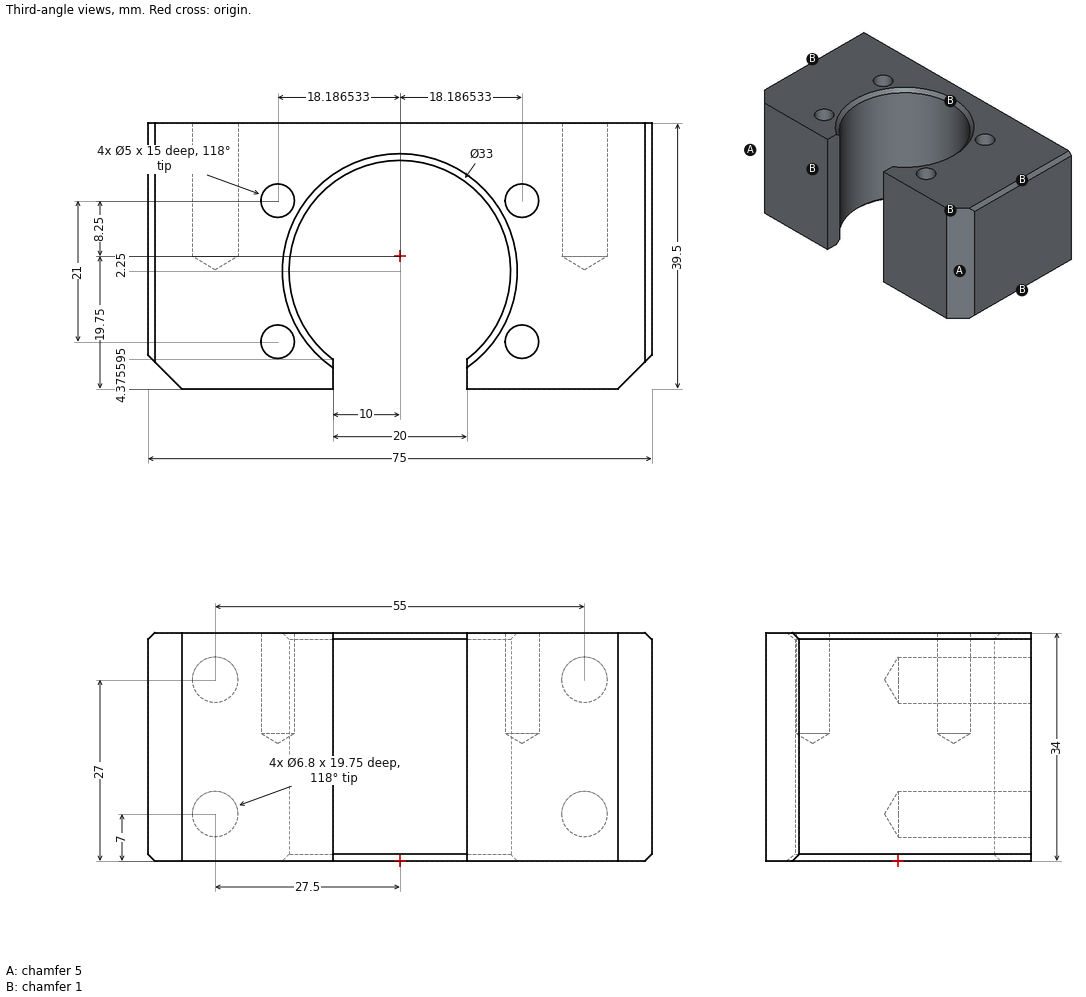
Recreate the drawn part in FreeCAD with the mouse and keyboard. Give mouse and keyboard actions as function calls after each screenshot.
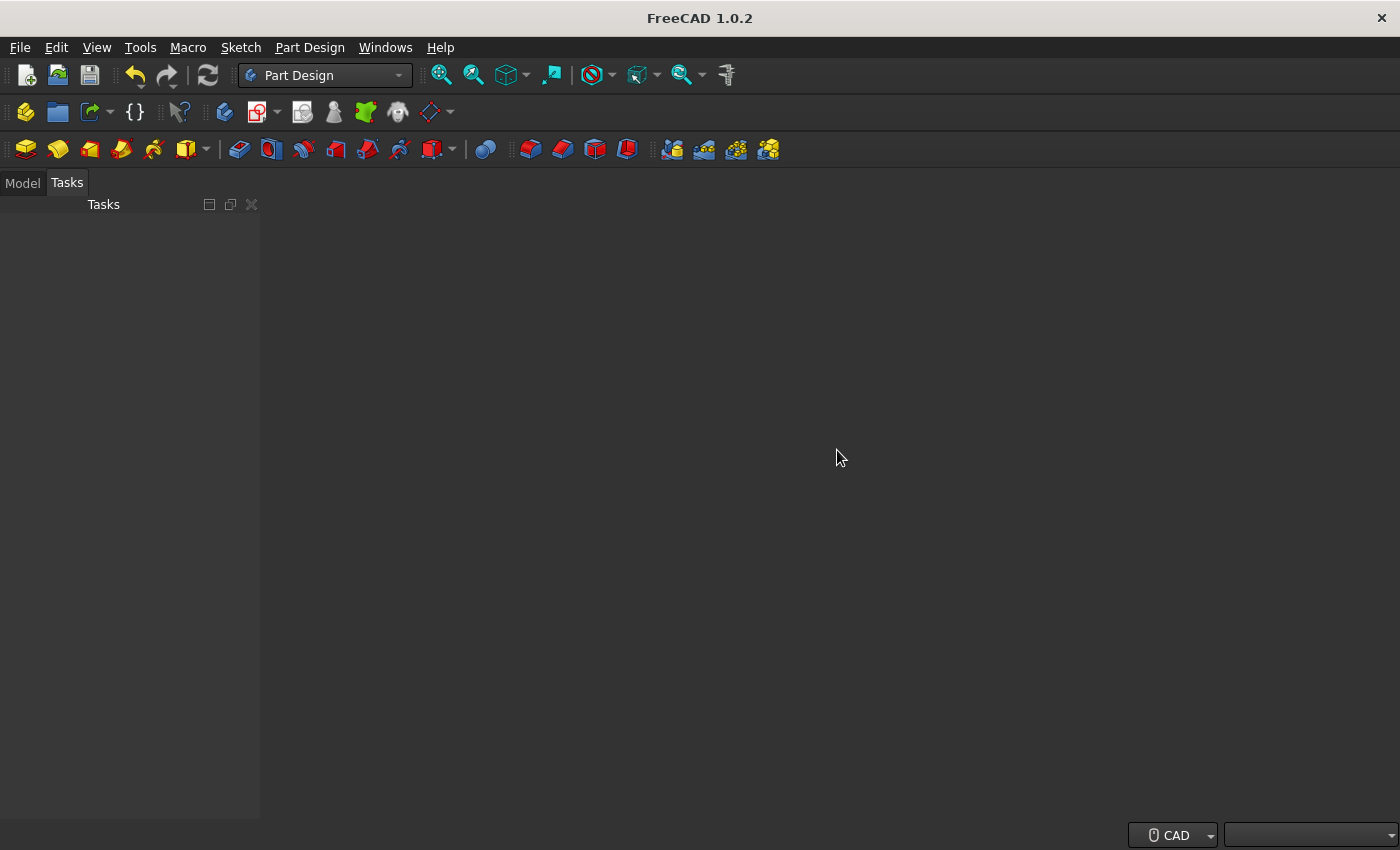
click(26, 76)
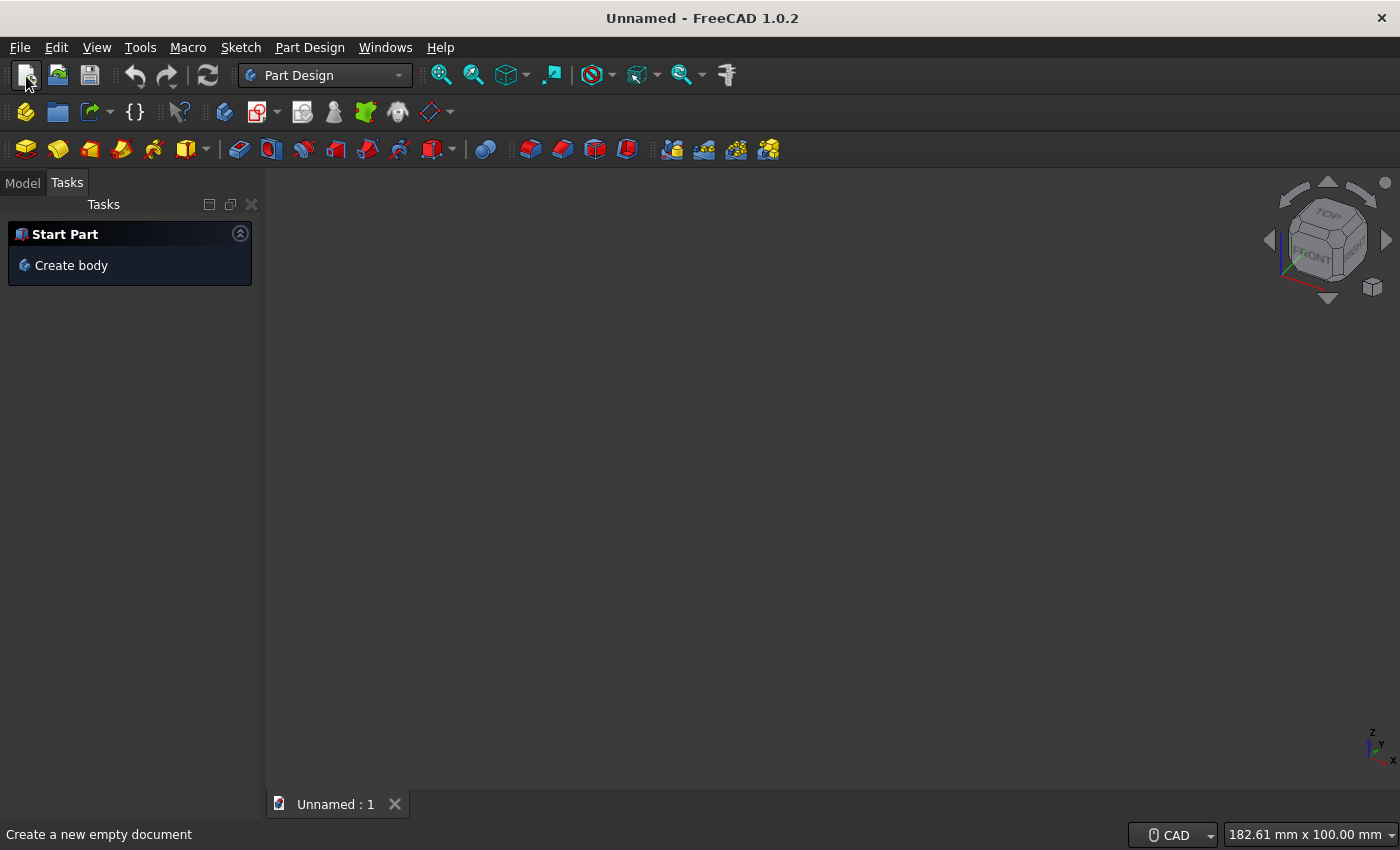
click(258, 112)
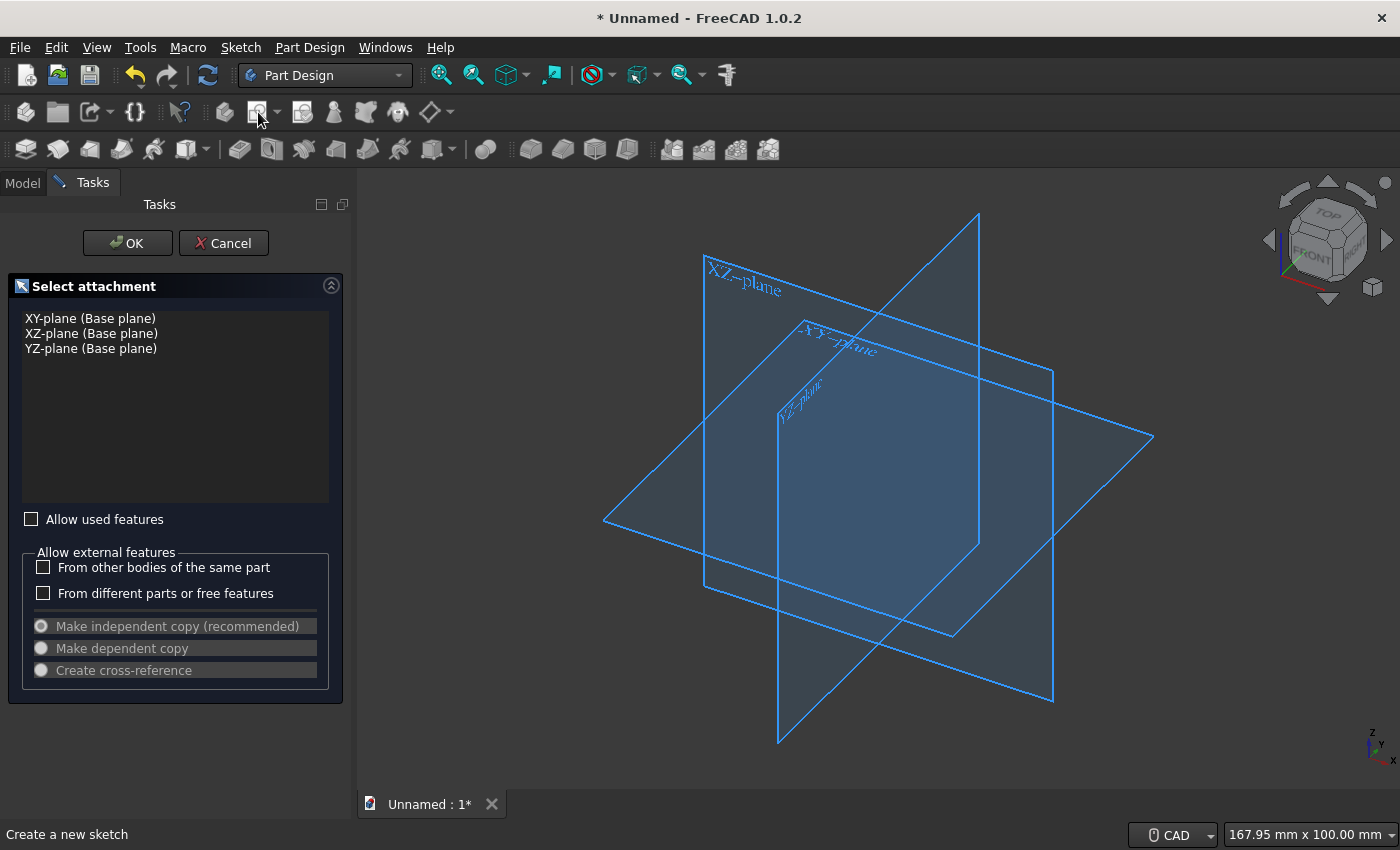
click(82, 318)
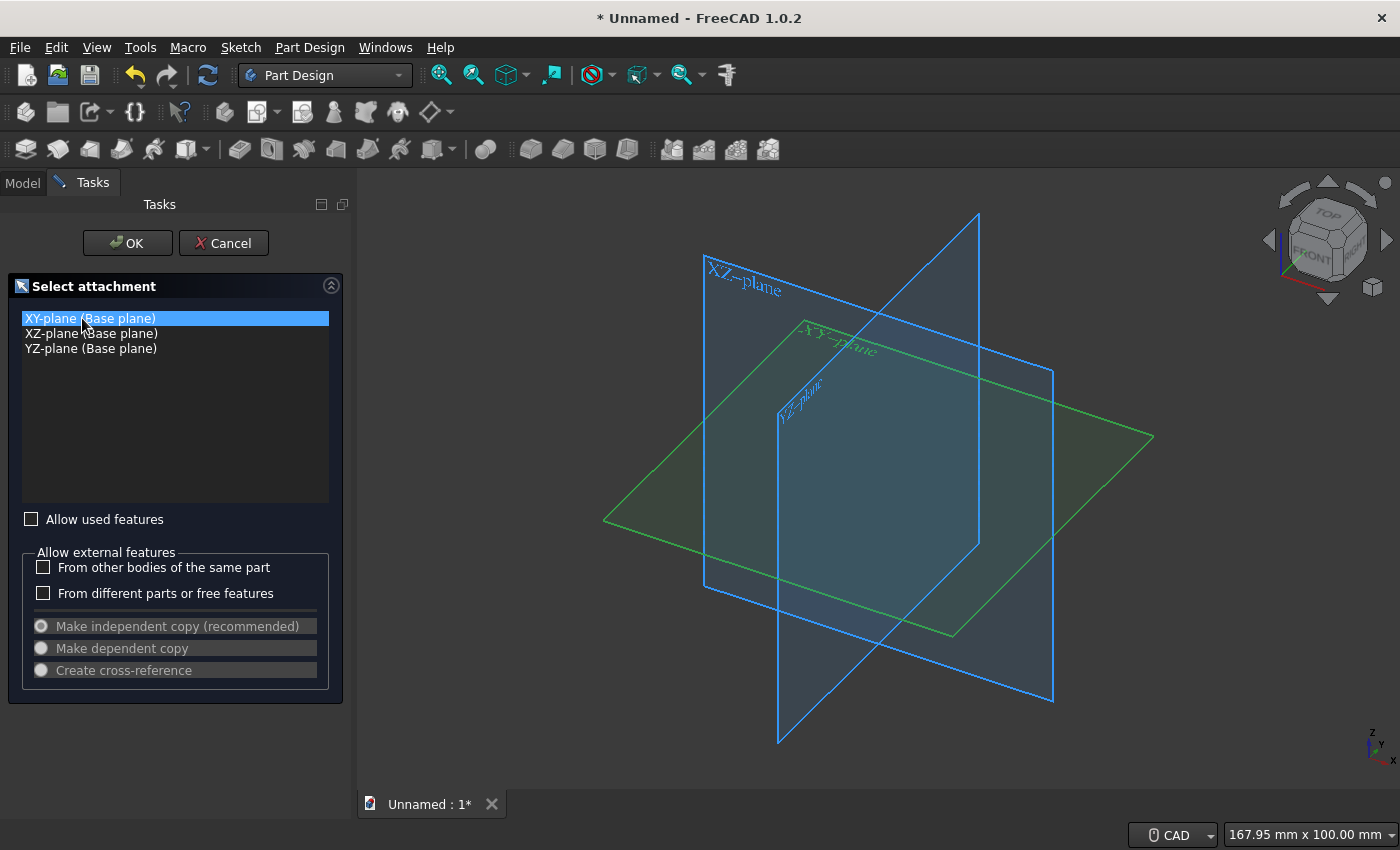
click(128, 243)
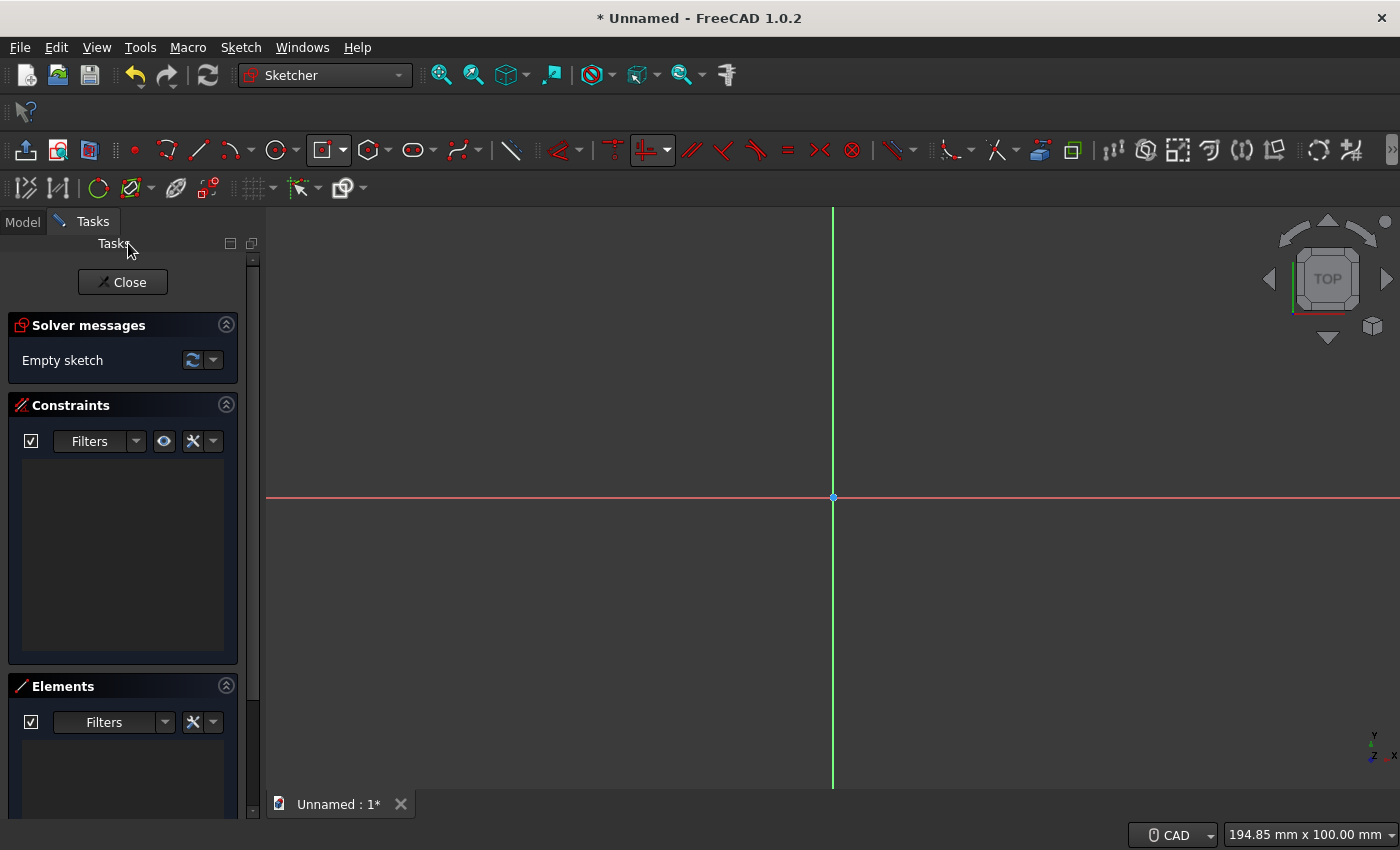
scroll(972, 498, up, 2)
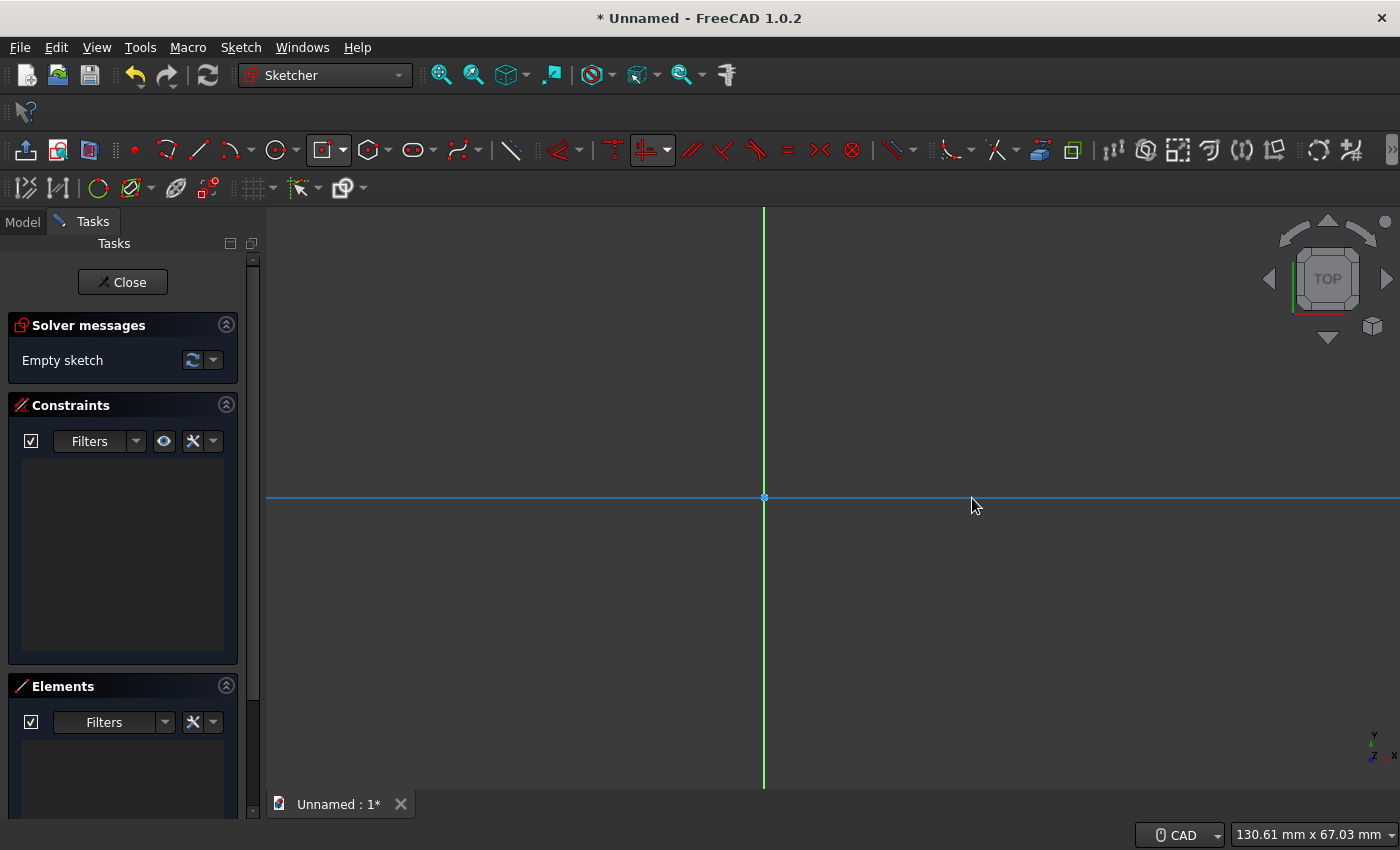
key(g)
key(v)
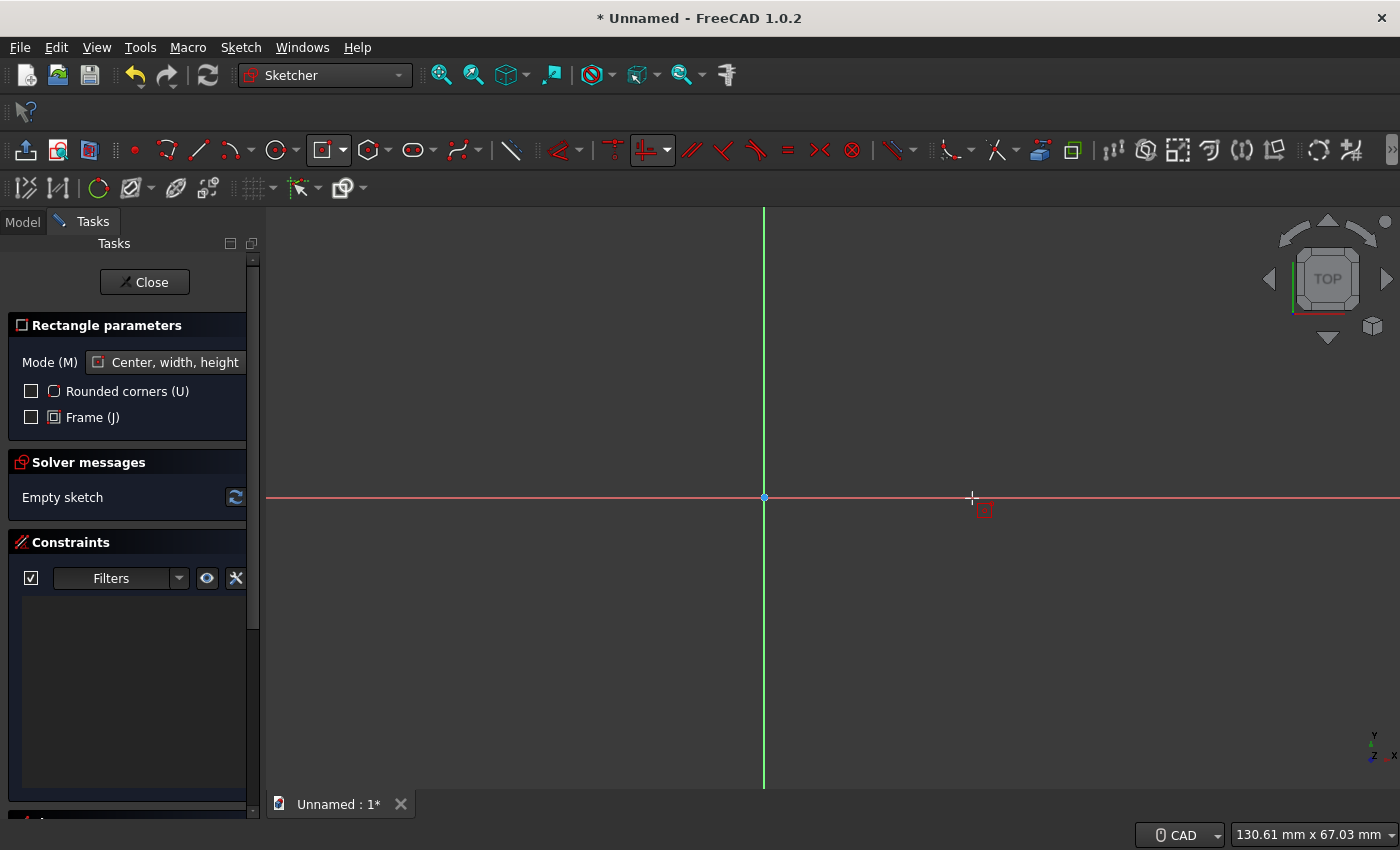
click(764, 498)
click(1090, 326)
key(Escape)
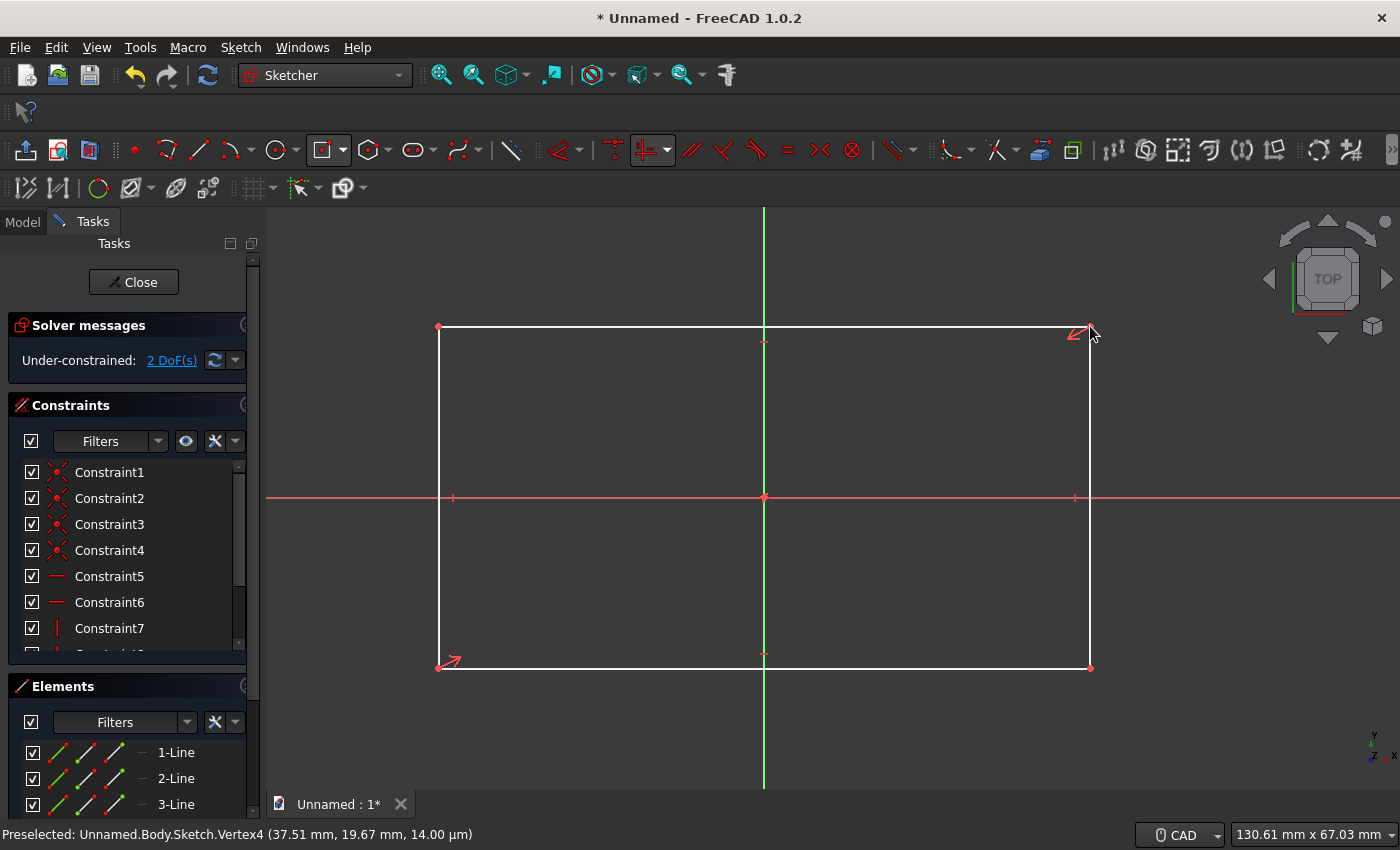
click(634, 669)